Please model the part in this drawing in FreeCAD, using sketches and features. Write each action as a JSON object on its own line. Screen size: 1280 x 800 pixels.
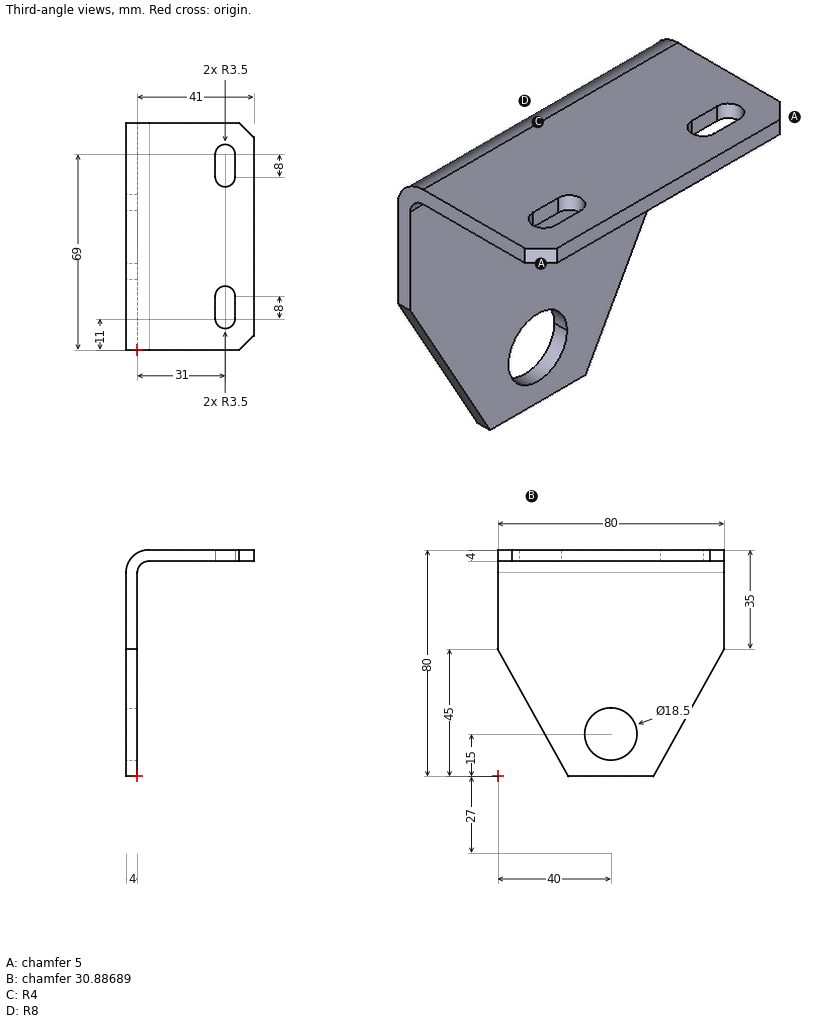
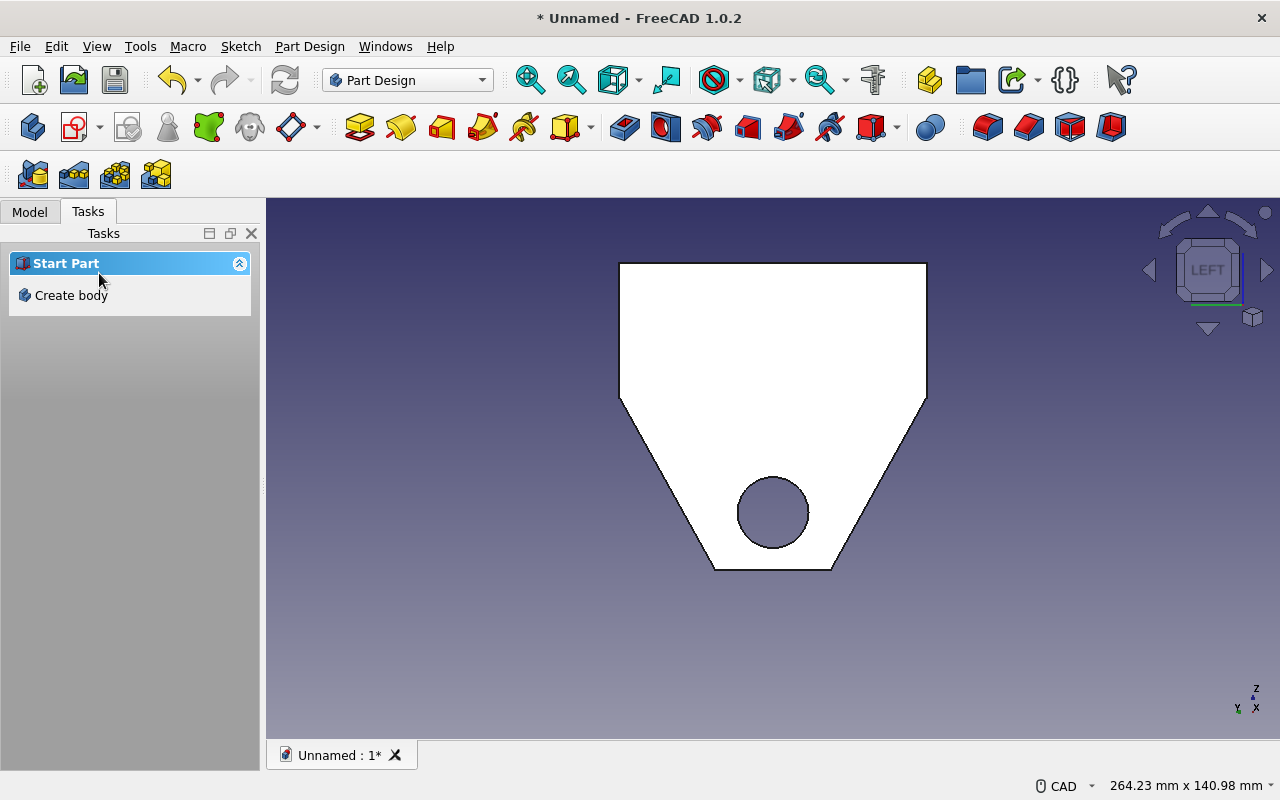
{"action": "key", "text": "v 3"}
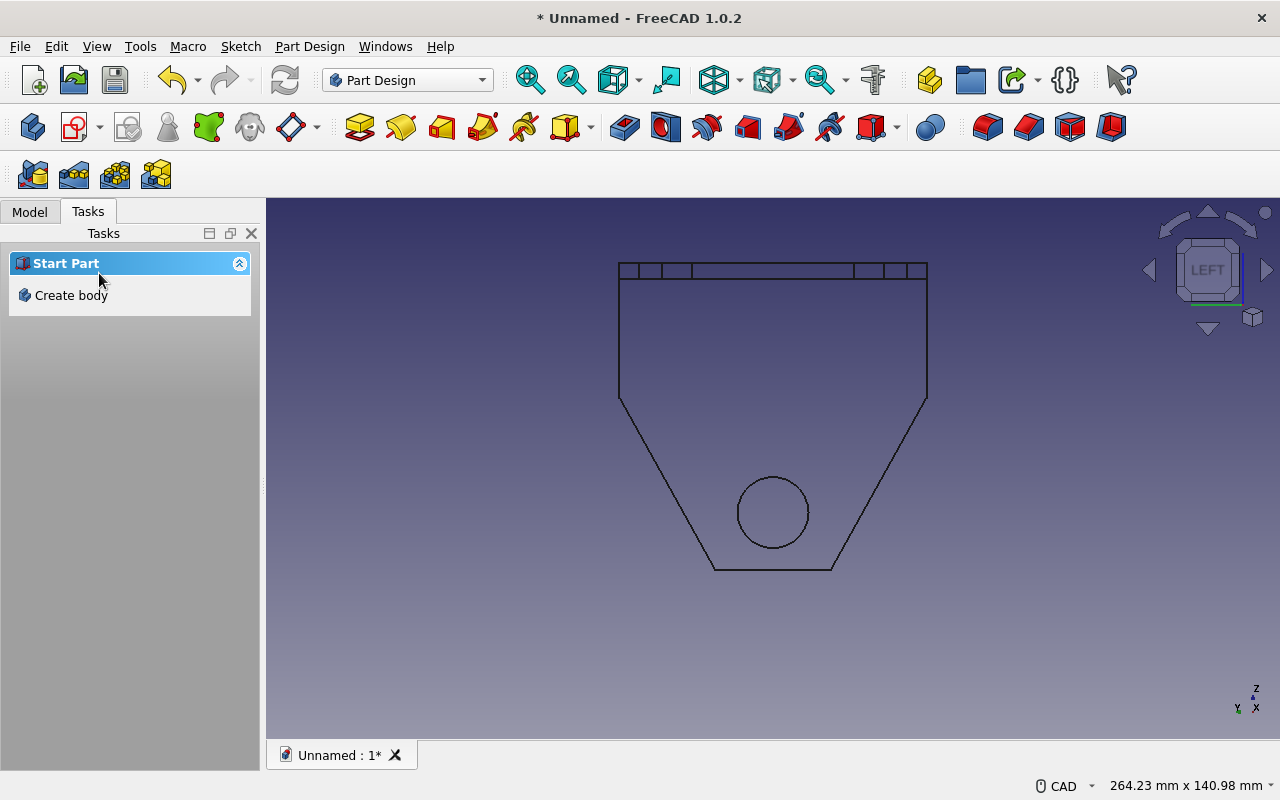
{"action": "key", "text": "0"}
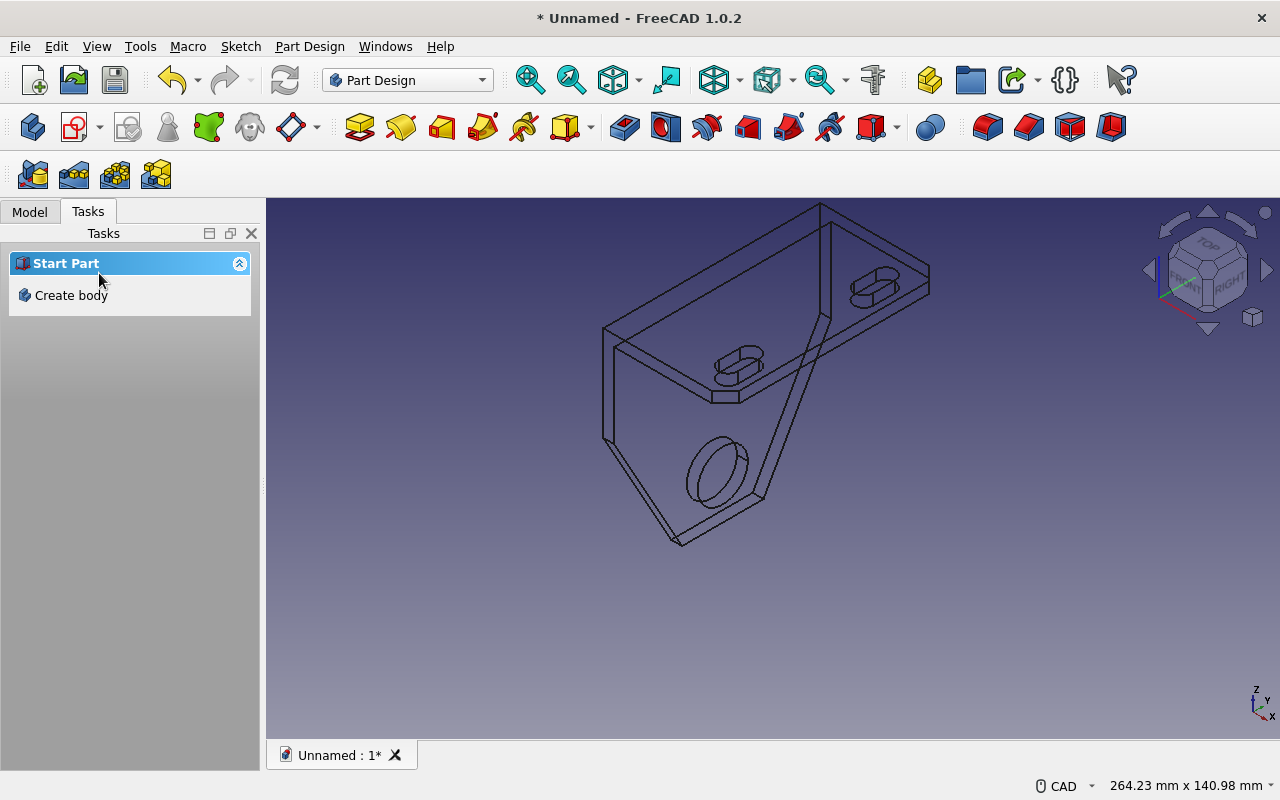
{"action": "left_click", "coordinate": [723, 283]}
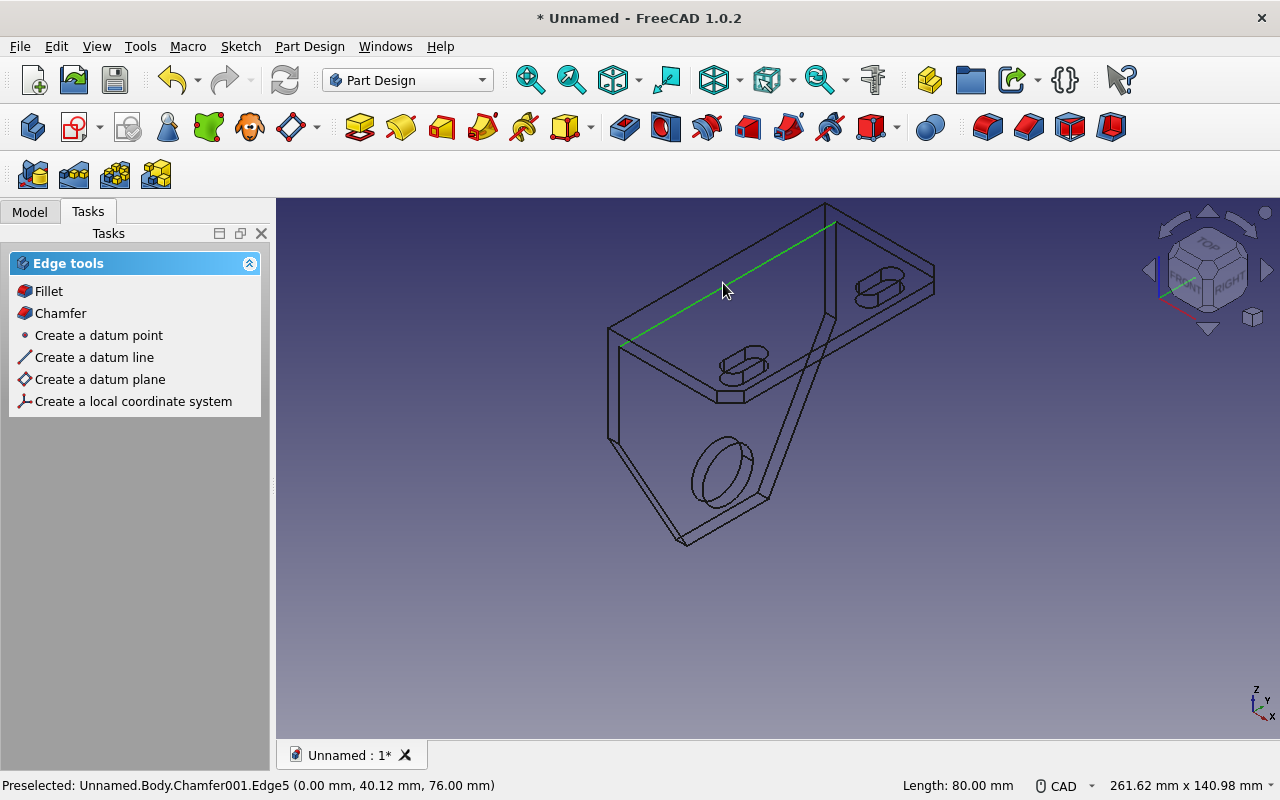
{"action": "key", "text": "v 1"}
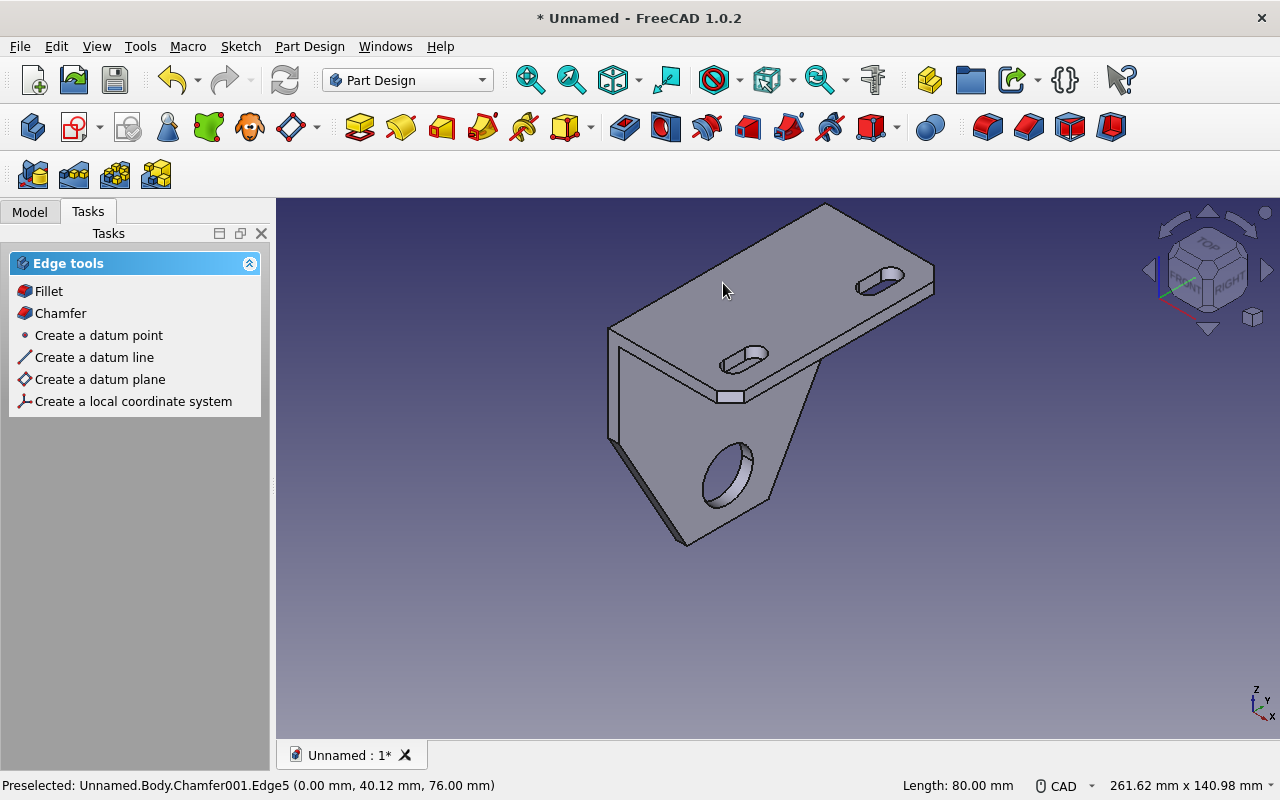
{"action": "left_click", "coordinate": [988, 128]}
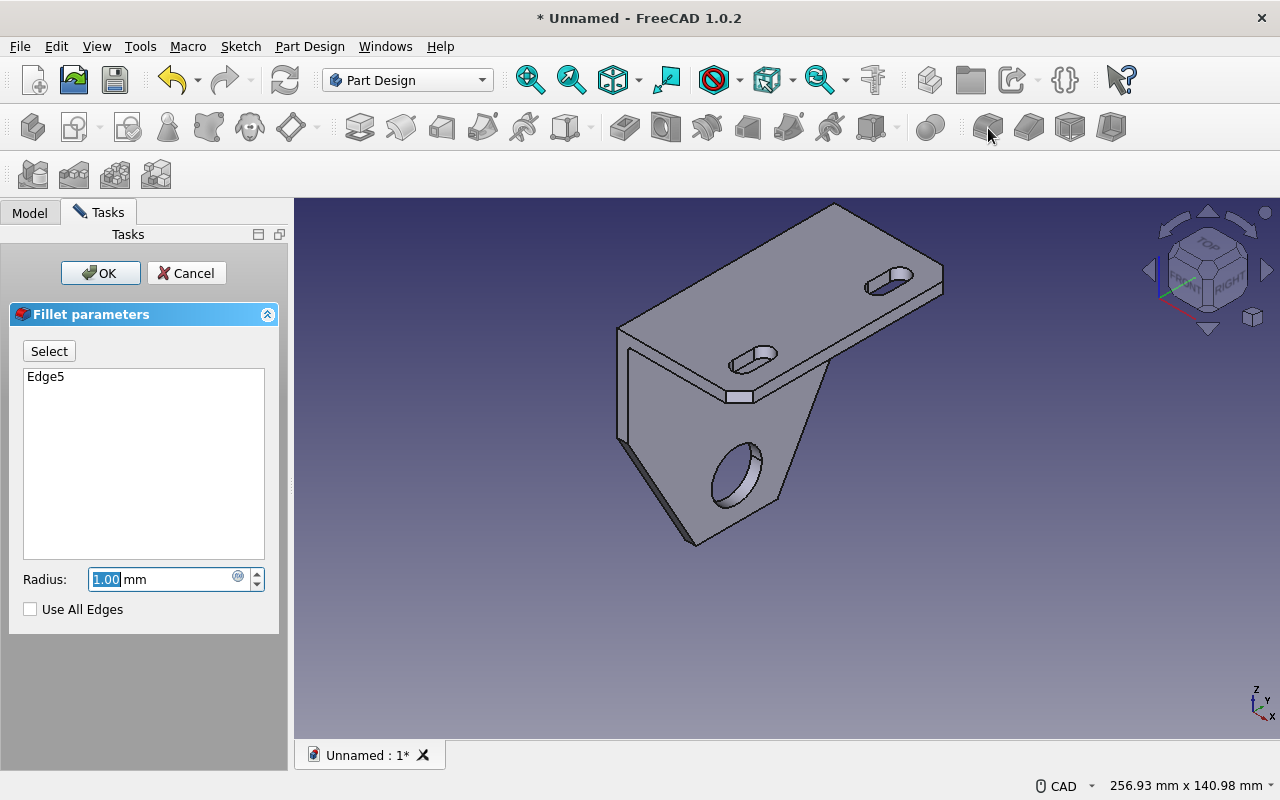
{"action": "type", "text": "4"}
{"action": "key", "text": "Tab"}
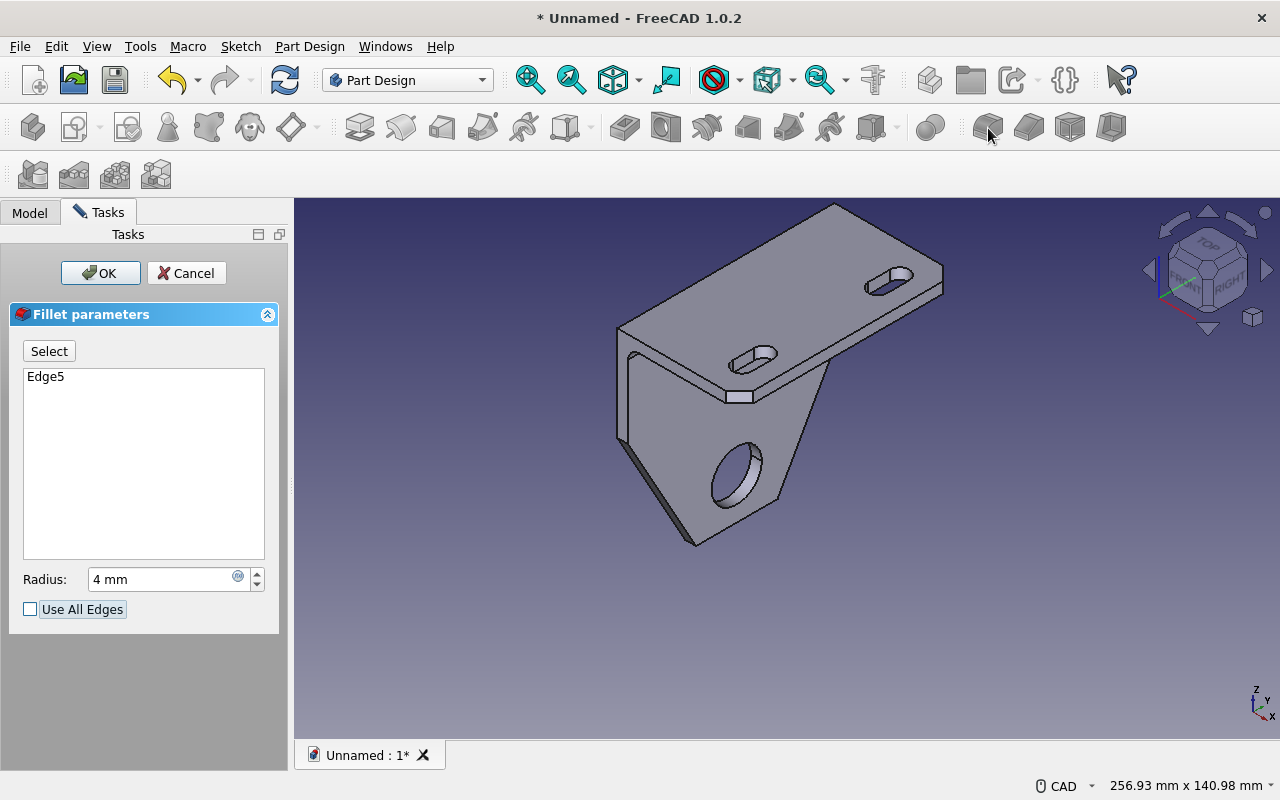
{"action": "left_click", "coordinate": [101, 273]}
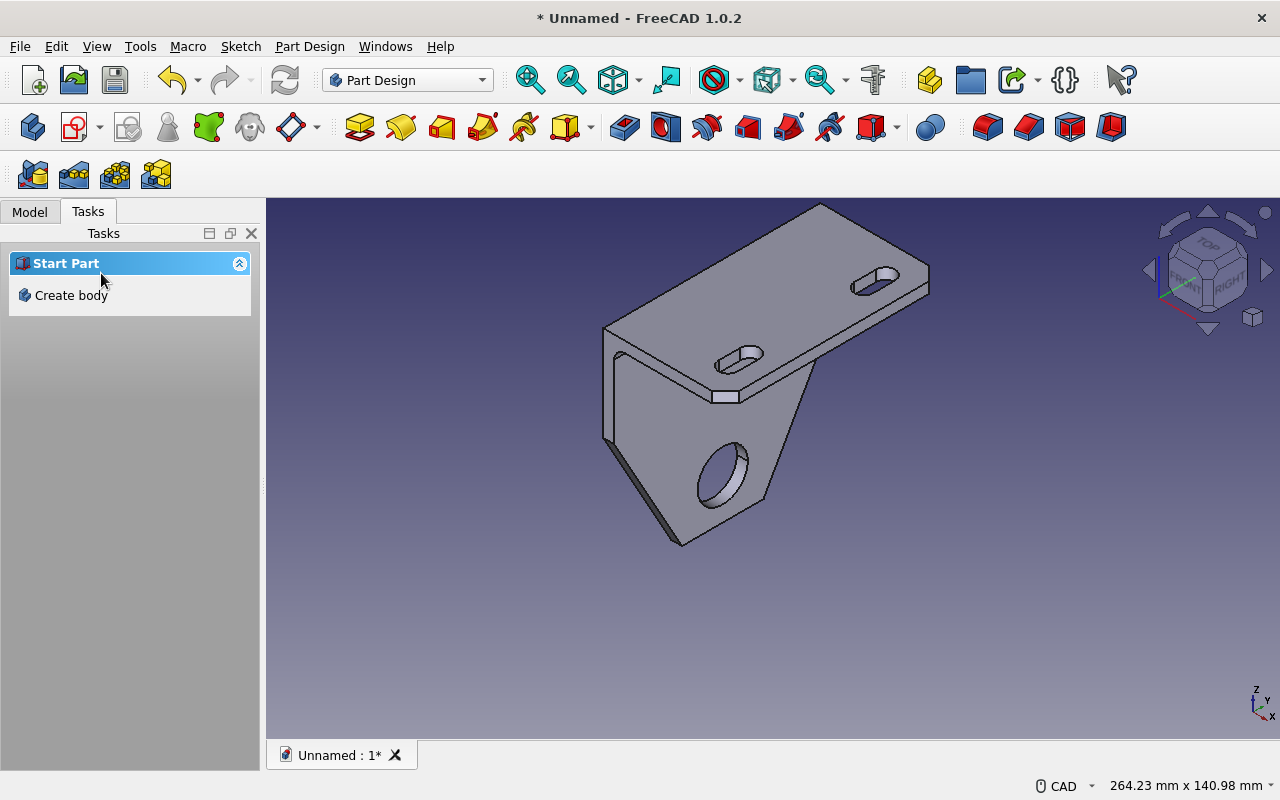
{"action": "key", "text": "2"}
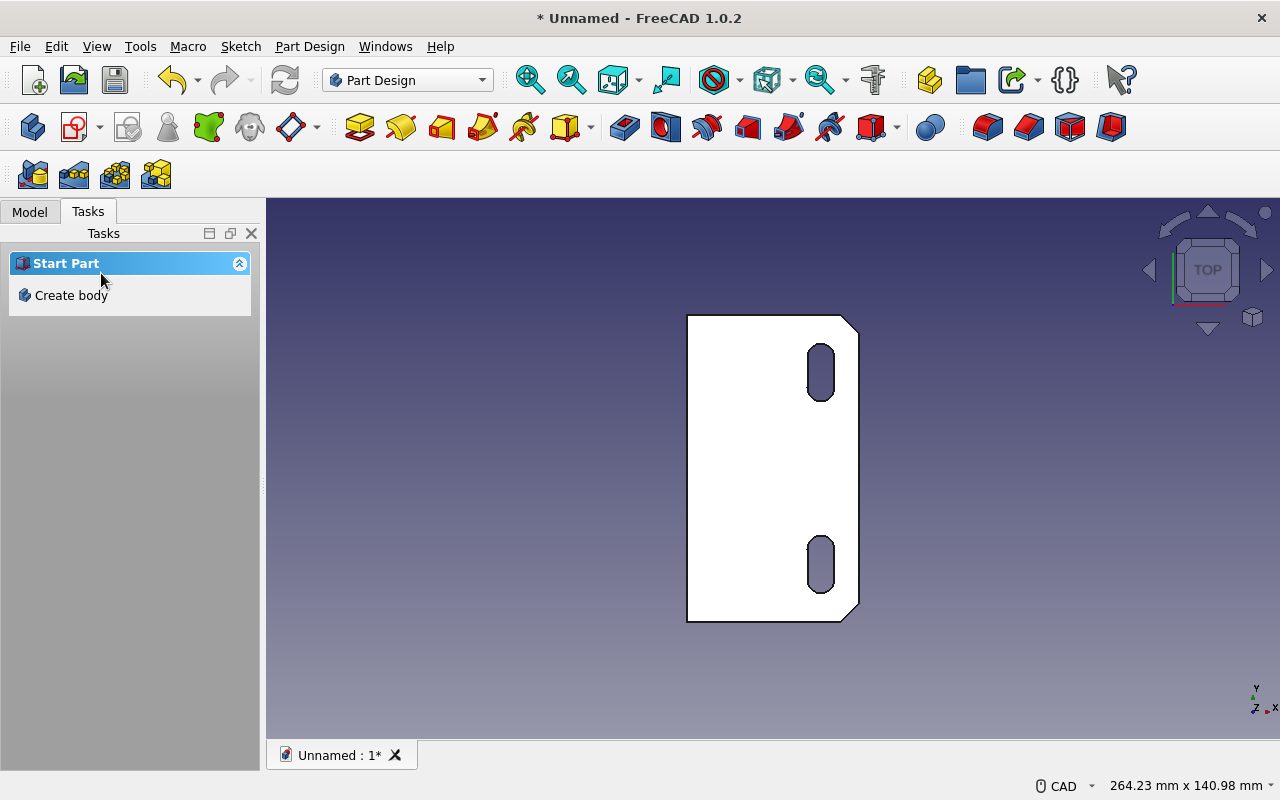
{"action": "left_click", "coordinate": [687, 467]}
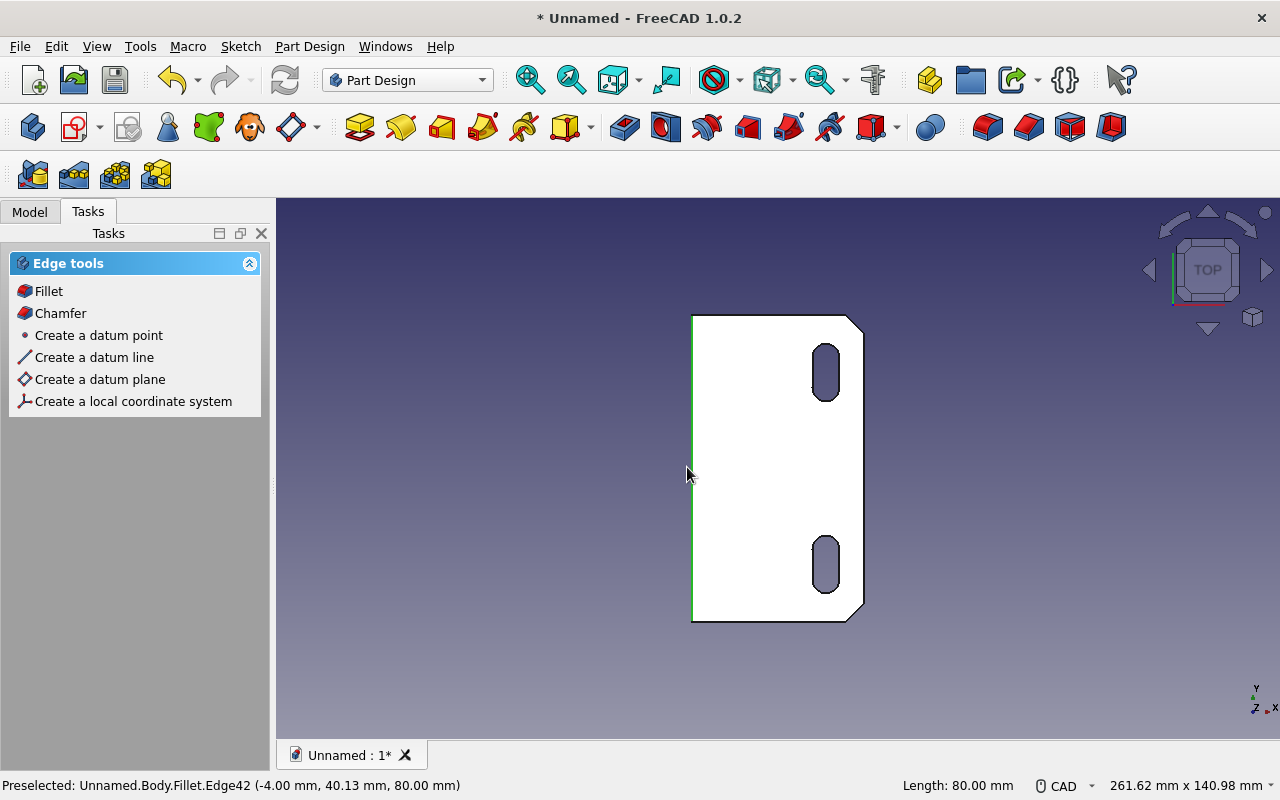
{"action": "left_click", "coordinate": [988, 128]}